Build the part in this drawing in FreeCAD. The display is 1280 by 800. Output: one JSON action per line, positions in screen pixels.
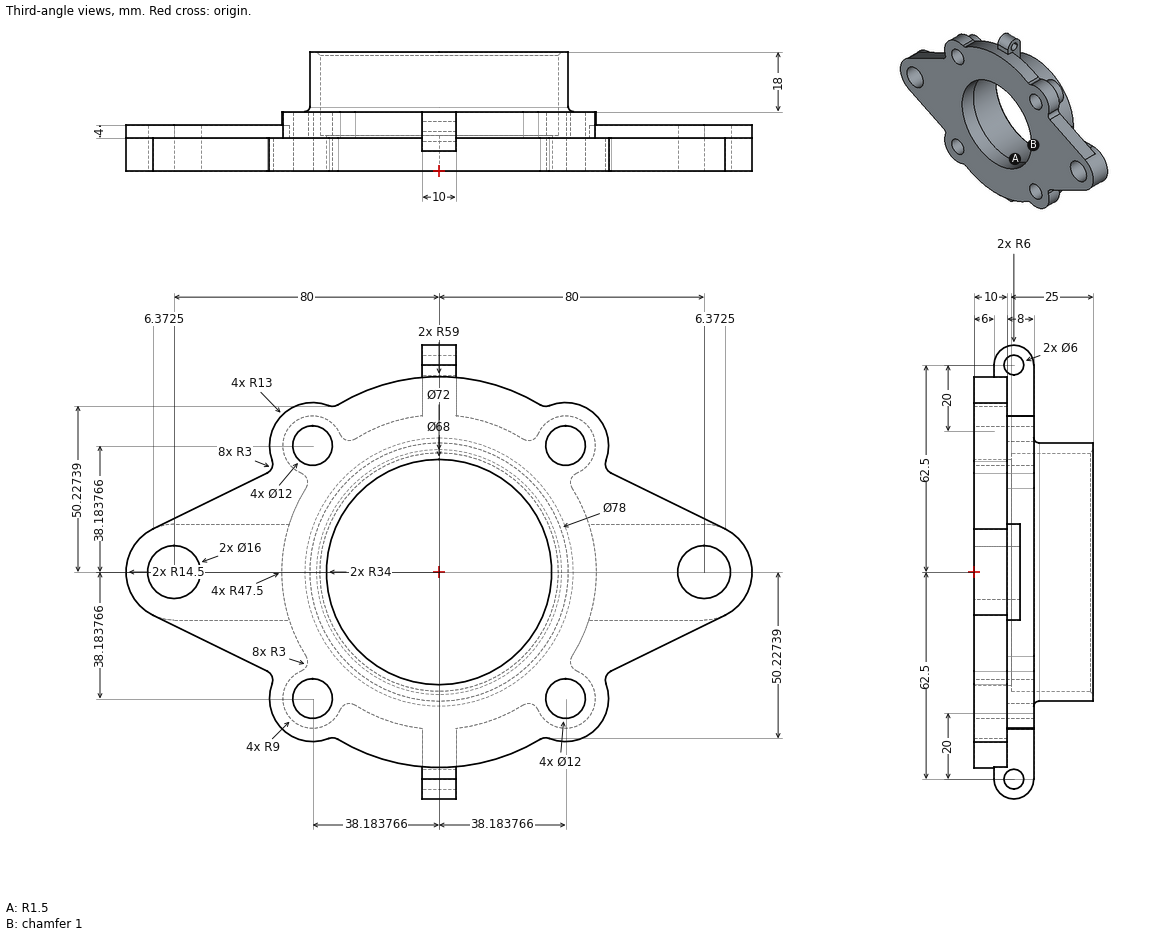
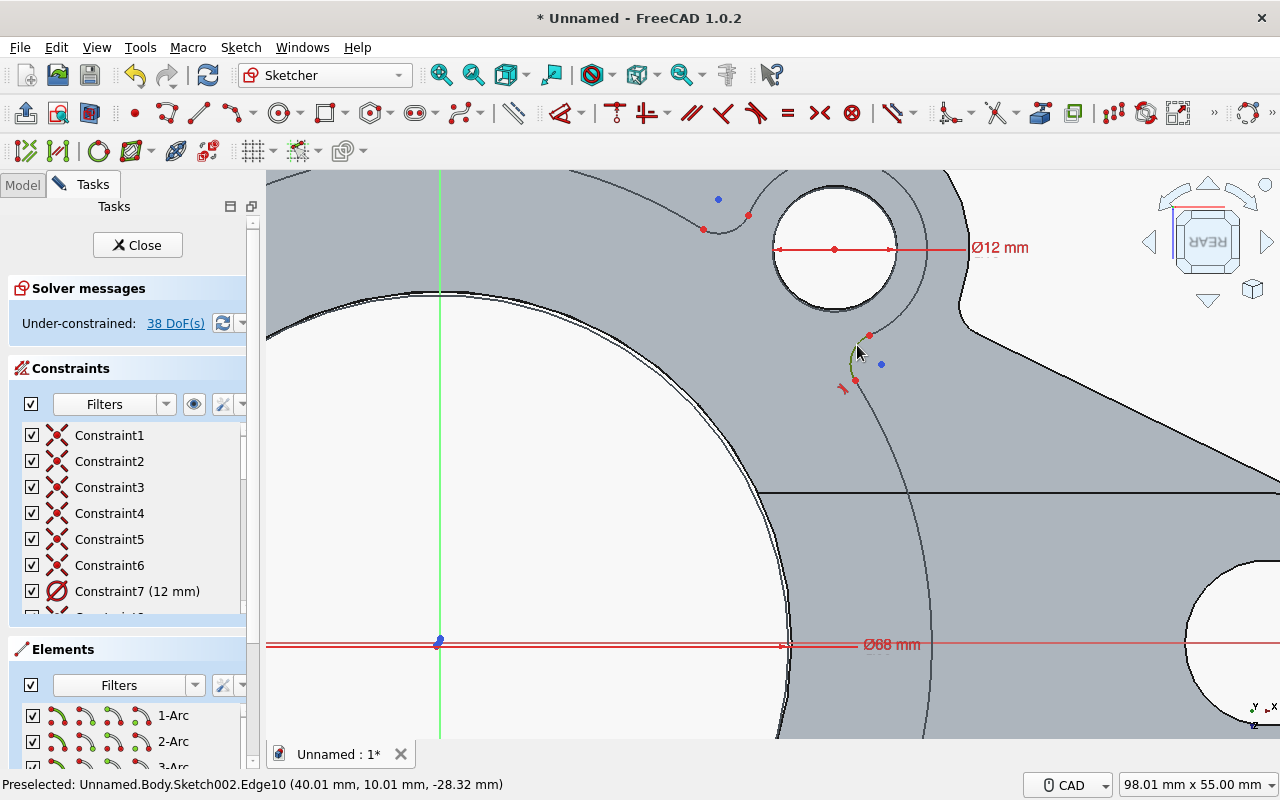
{"action": "left_click", "coordinate": [927, 250]}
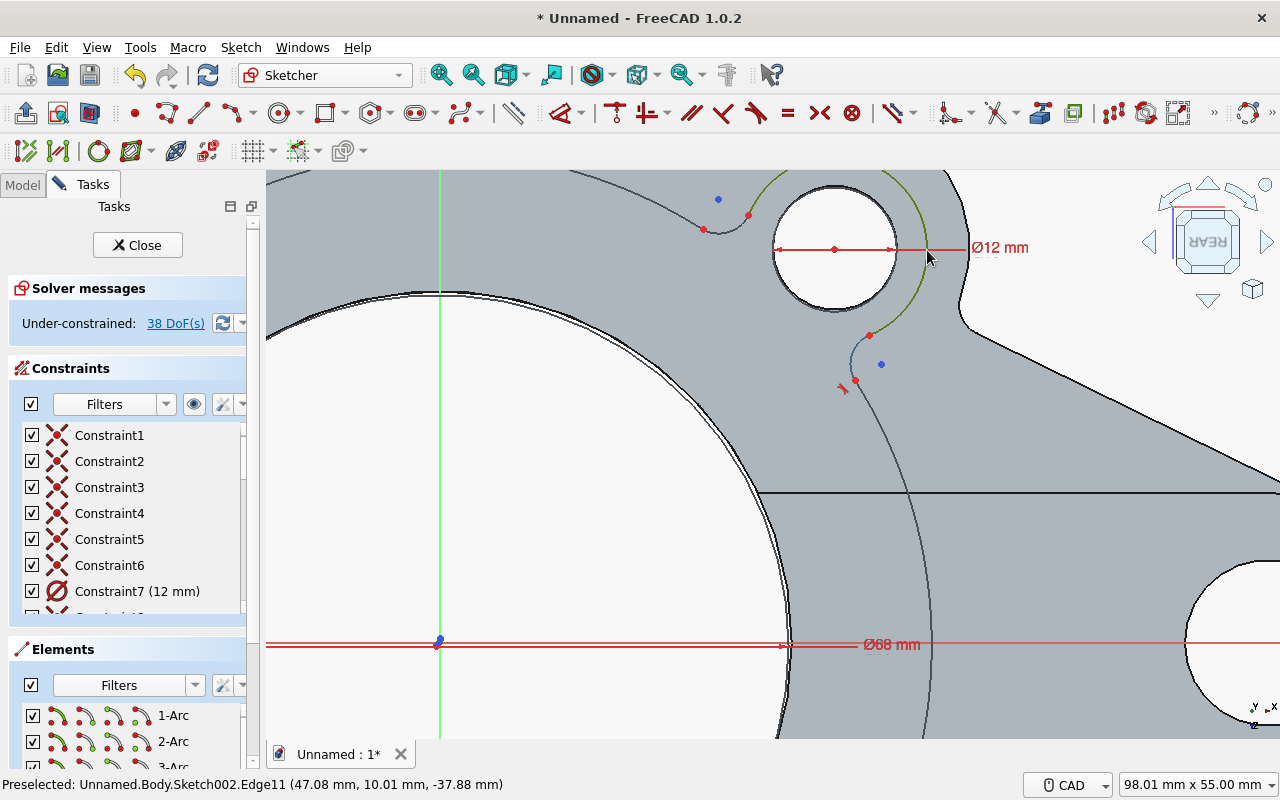
{"action": "left_click", "coordinate": [756, 114]}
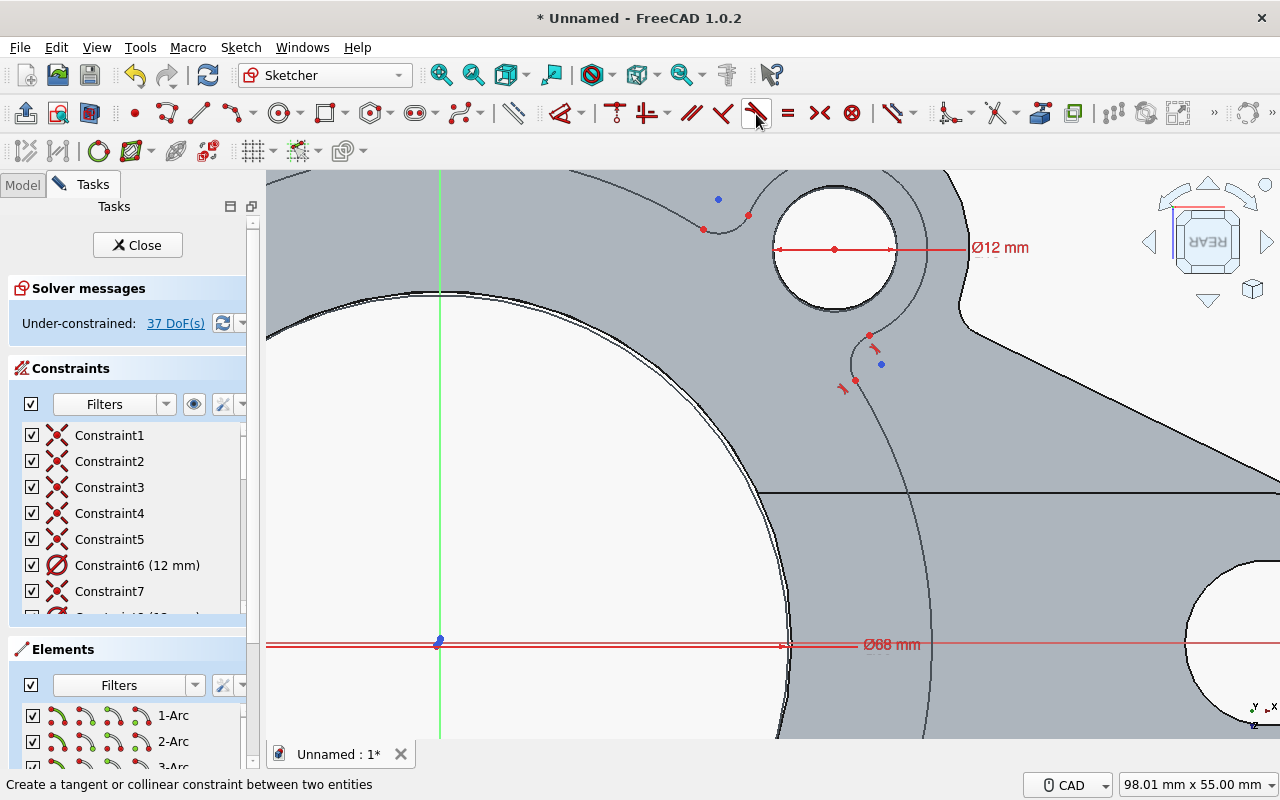
{"action": "left_click", "coordinate": [927, 250]}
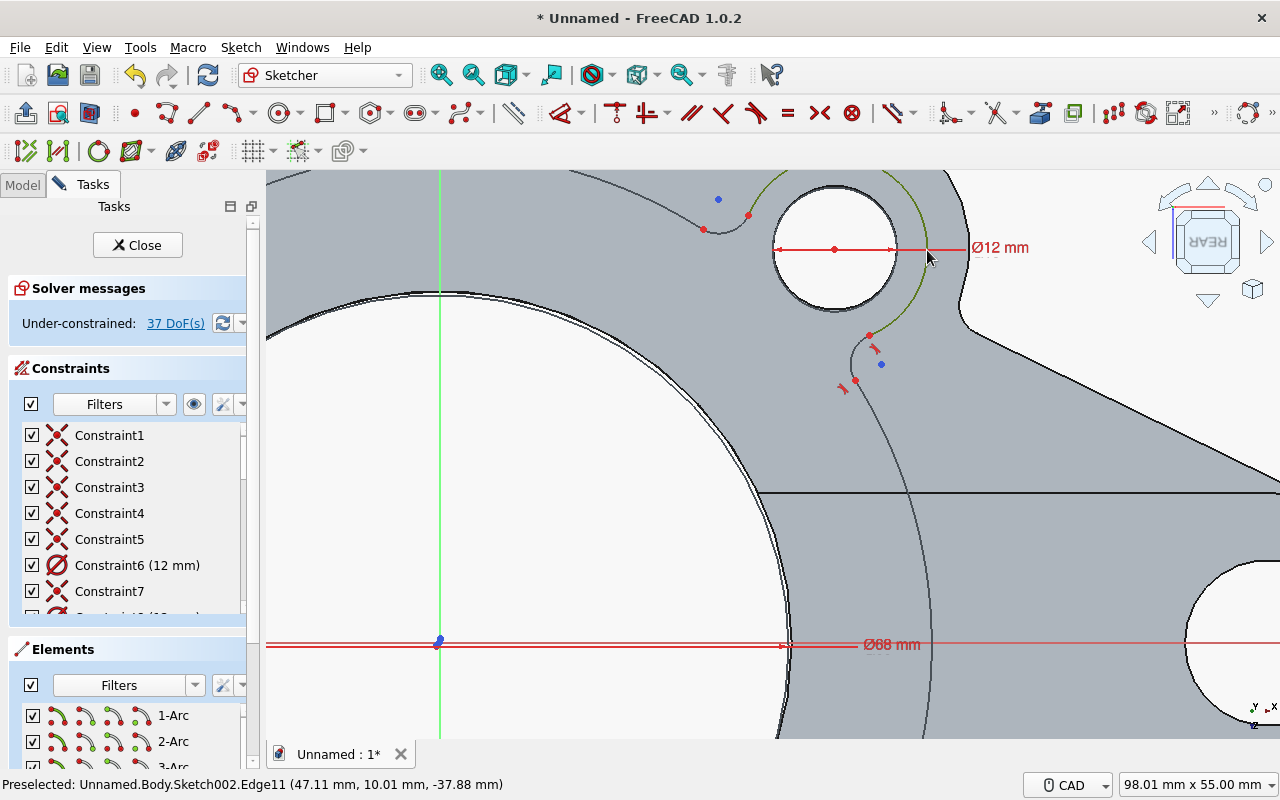
{"action": "left_click", "coordinate": [719, 234]}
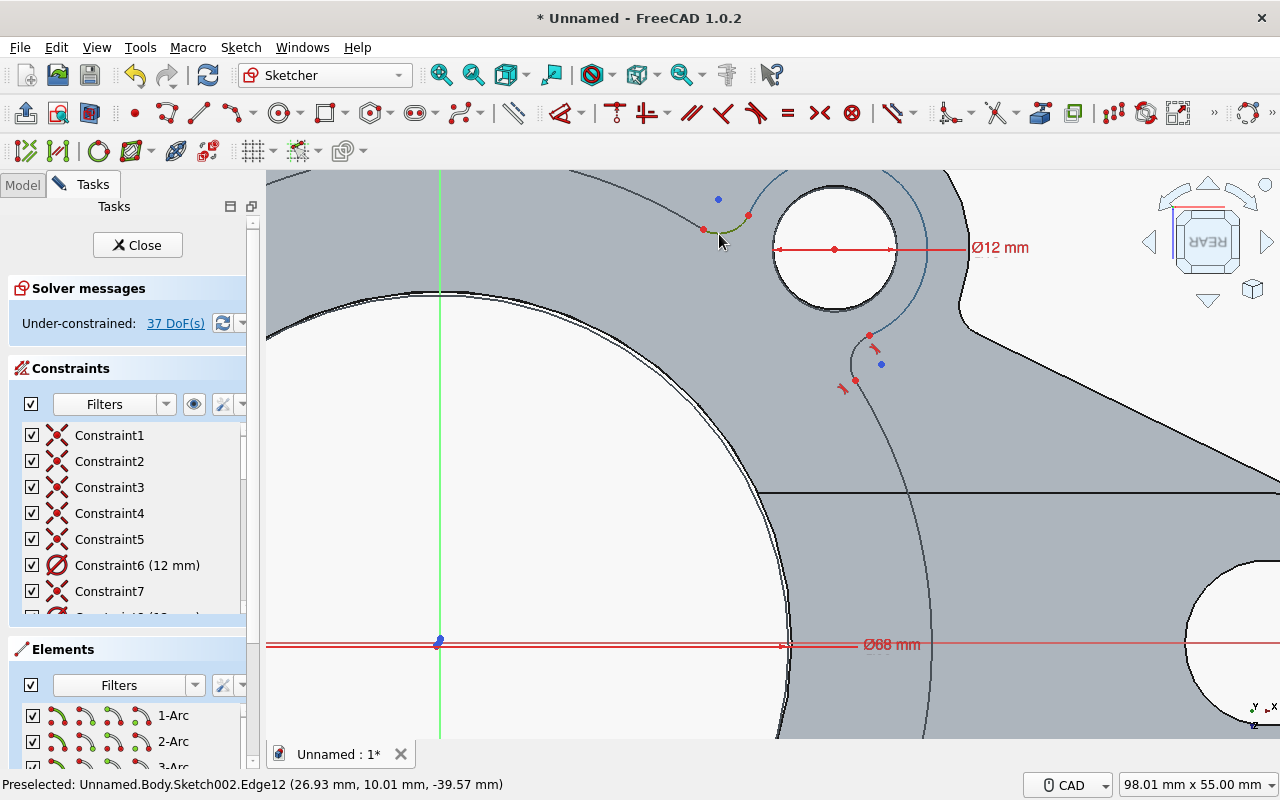
{"action": "left_click", "coordinate": [756, 114]}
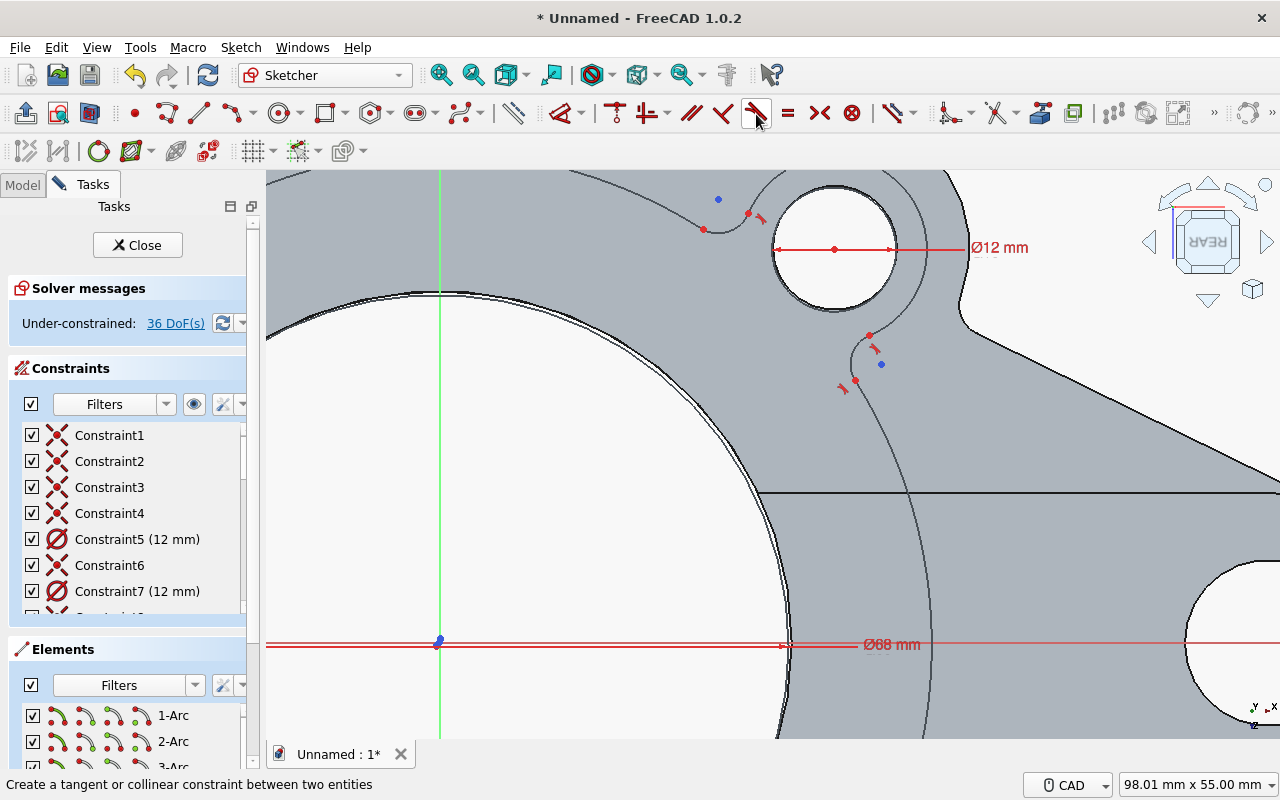
{"action": "left_click", "coordinate": [719, 233]}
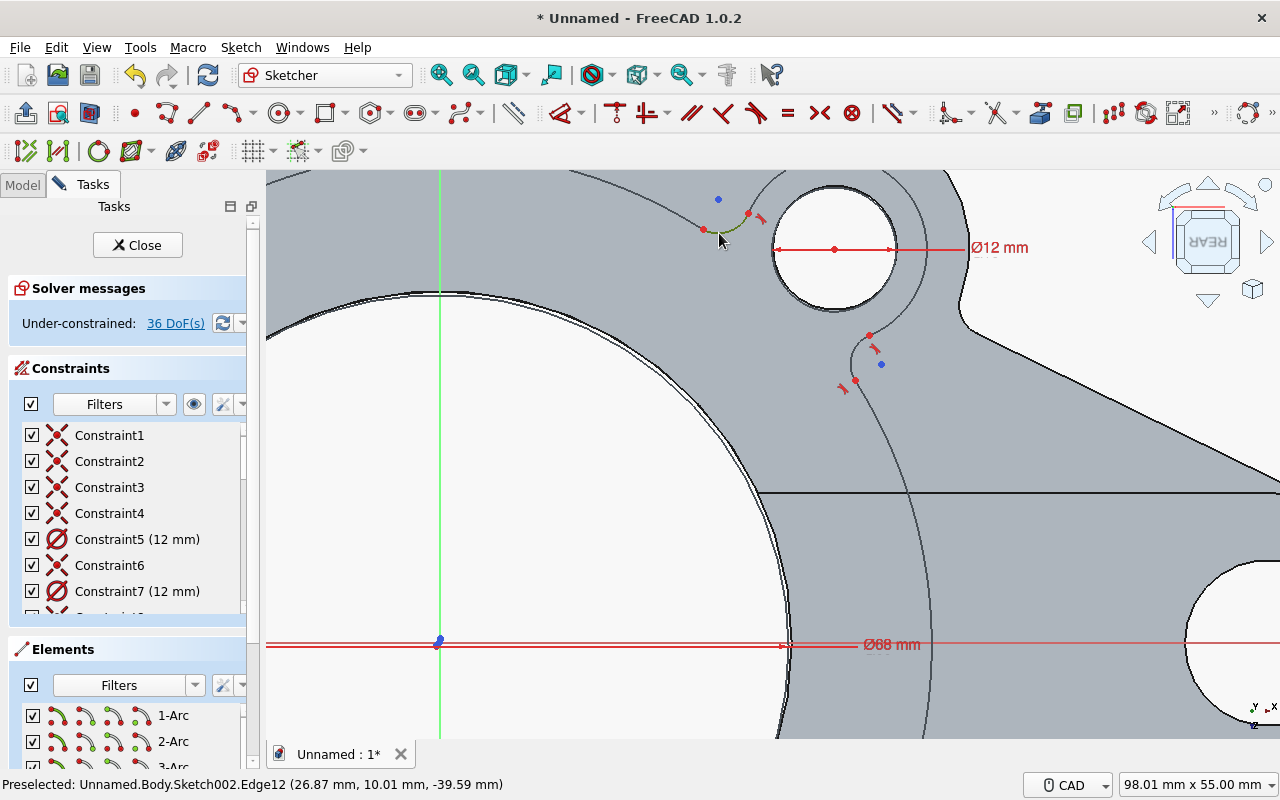
{"action": "scroll", "coordinate": [858, 345], "scroll_direction": "down", "scroll_amount": 5}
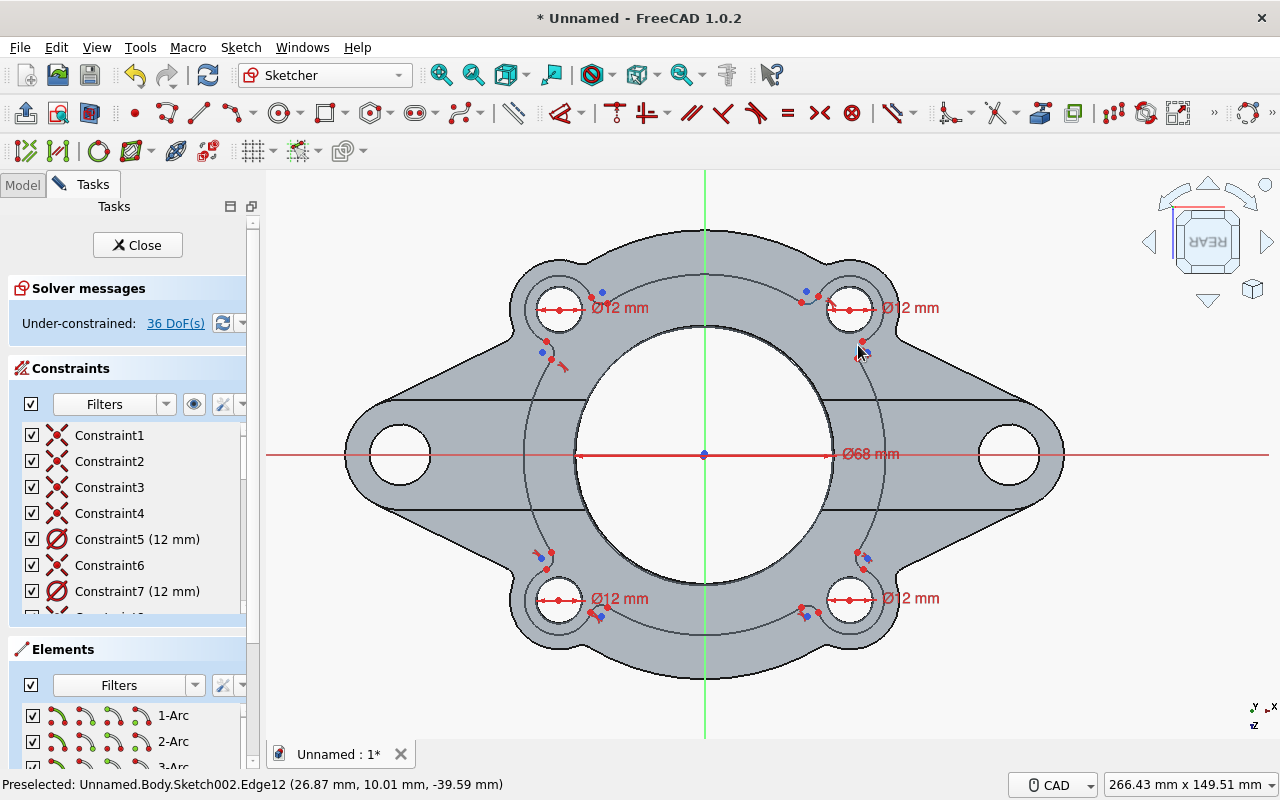
{"action": "left_click", "coordinate": [745, 279]}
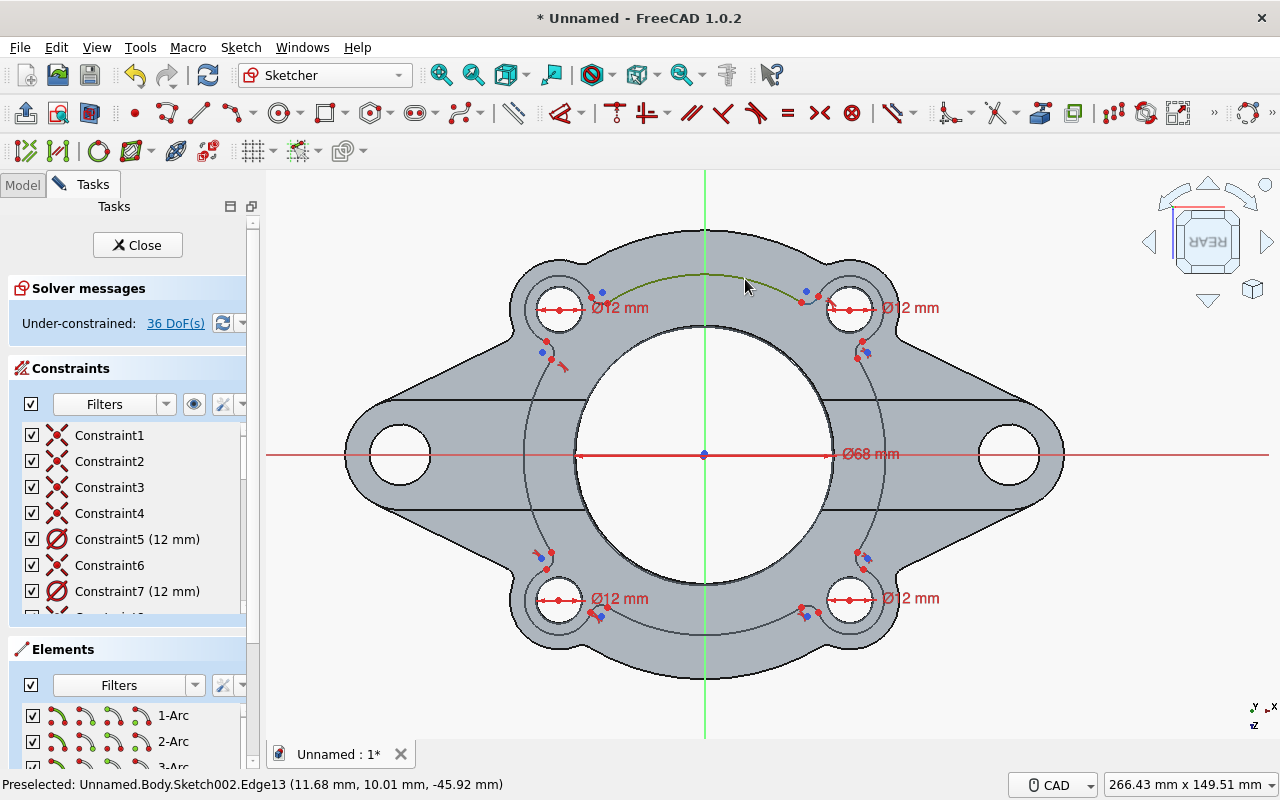
{"action": "left_click", "coordinate": [756, 114]}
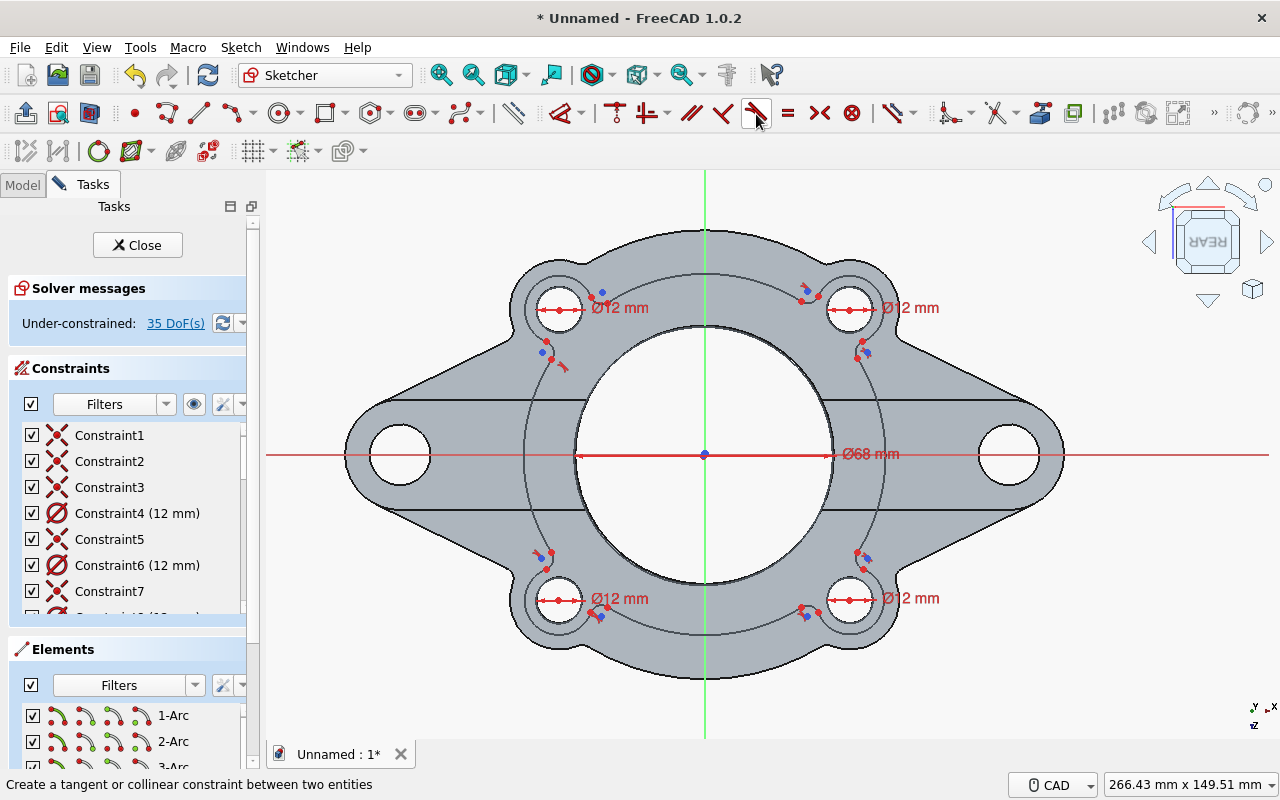
{"action": "left_click", "coordinate": [745, 278]}